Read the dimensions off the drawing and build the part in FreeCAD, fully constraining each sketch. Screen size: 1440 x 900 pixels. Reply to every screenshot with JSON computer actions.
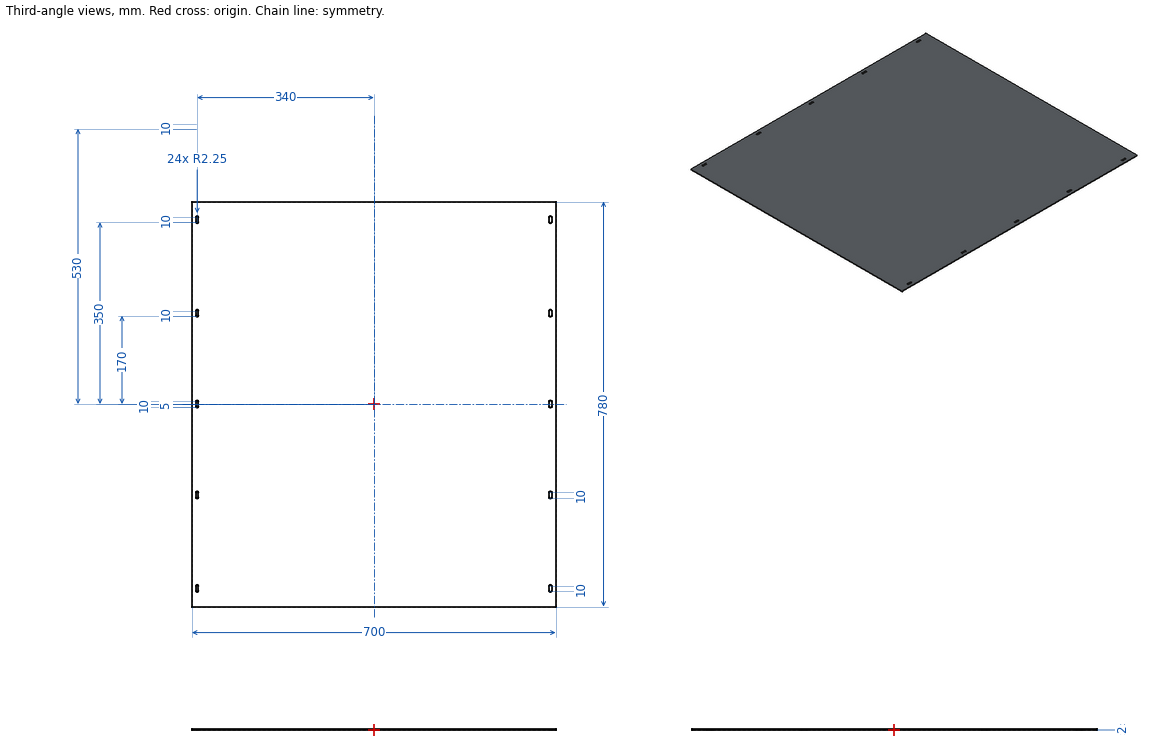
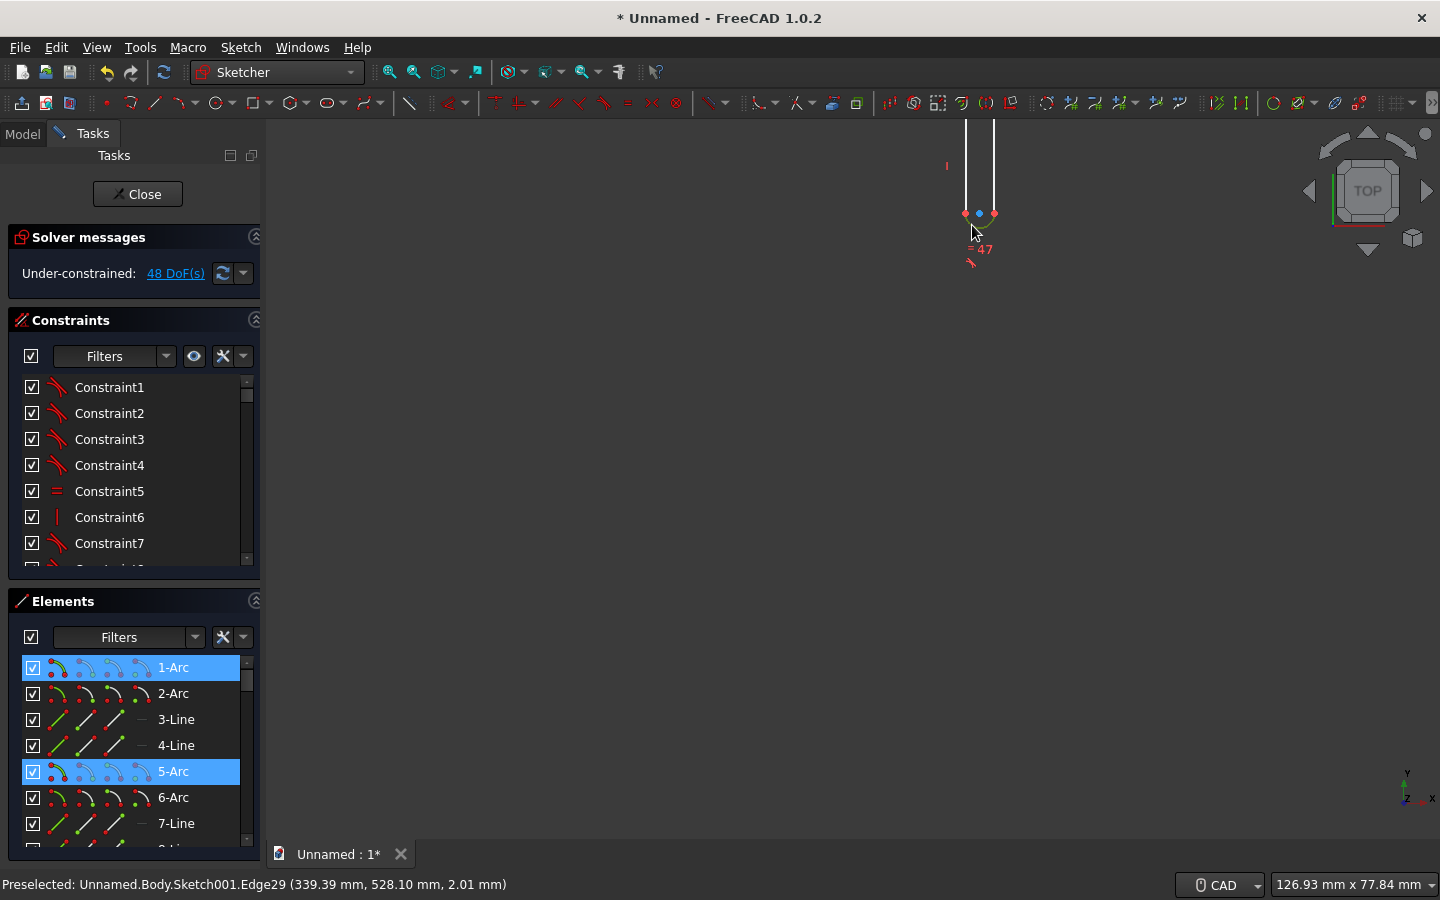
{"action": "scroll", "coordinate": [976, 233], "scroll_direction": "down", "scroll_amount": 14}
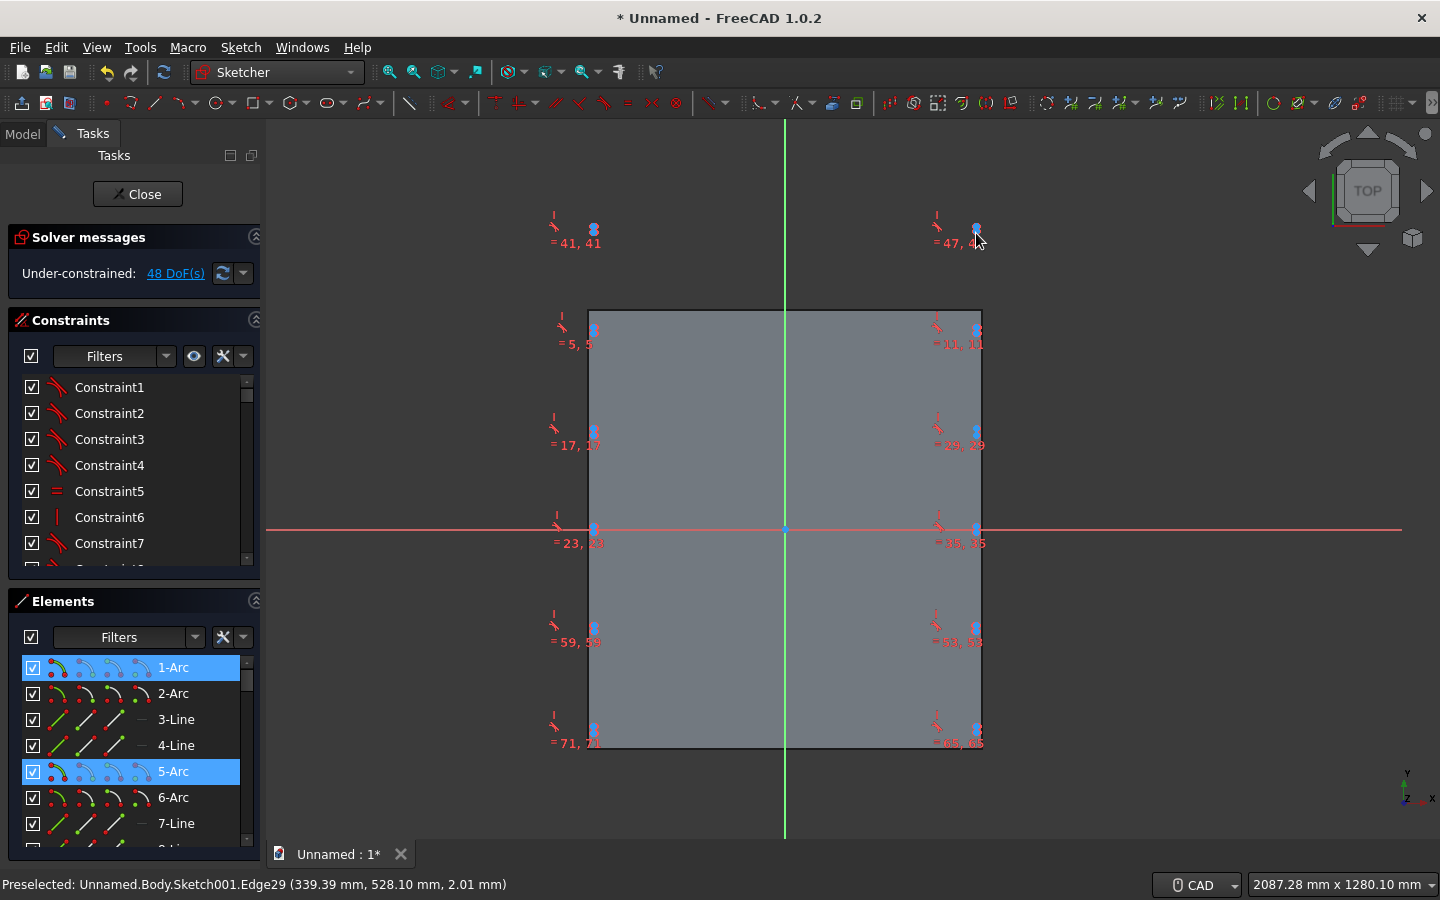
{"action": "scroll", "coordinate": [976, 633], "scroll_direction": "up", "scroll_amount": 13}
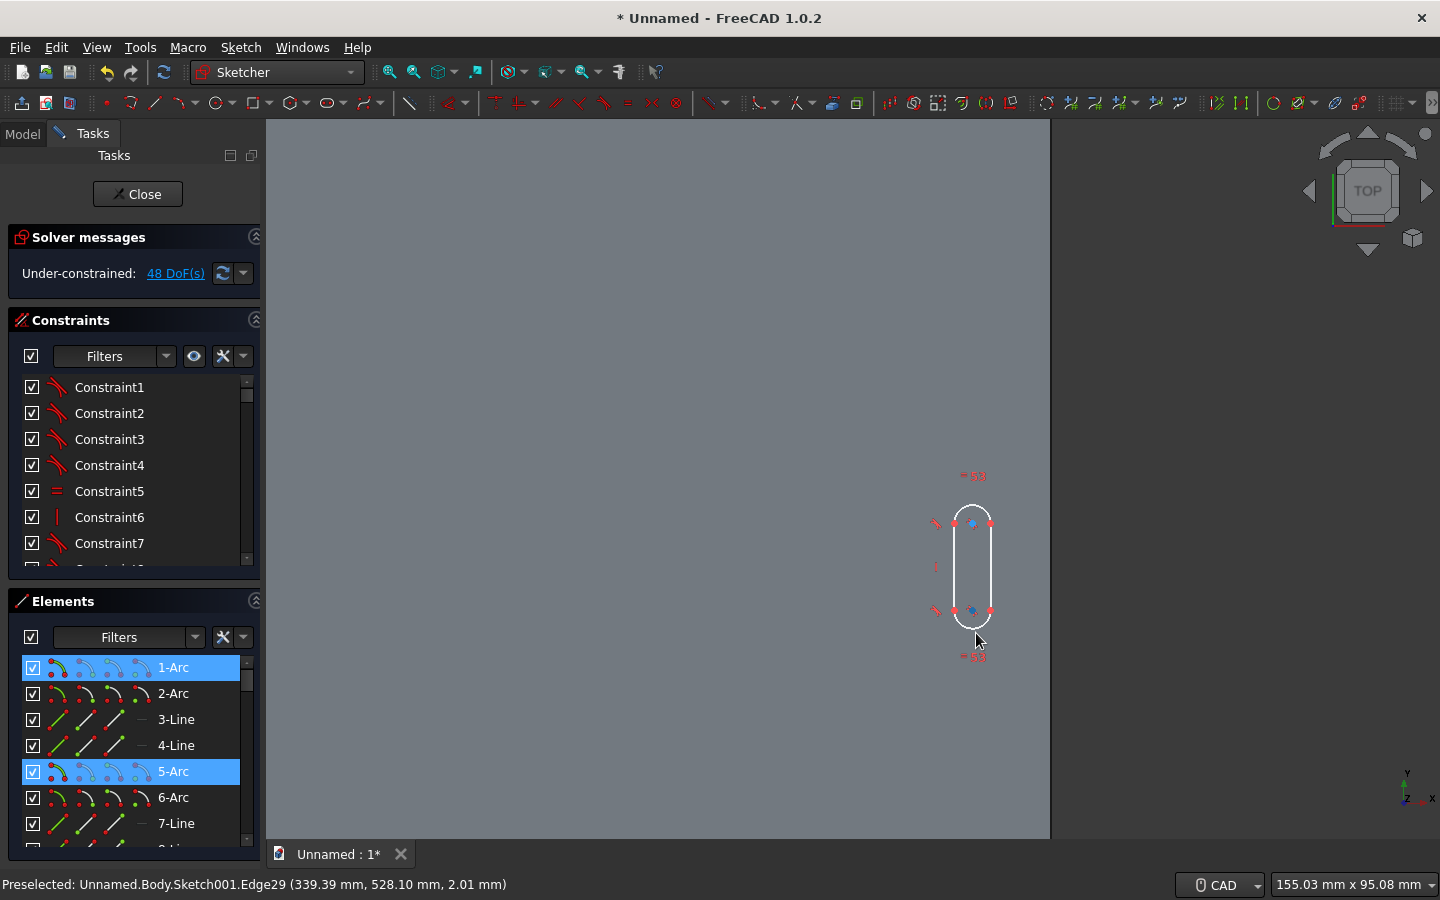
{"action": "left_click", "coordinate": [962, 625]}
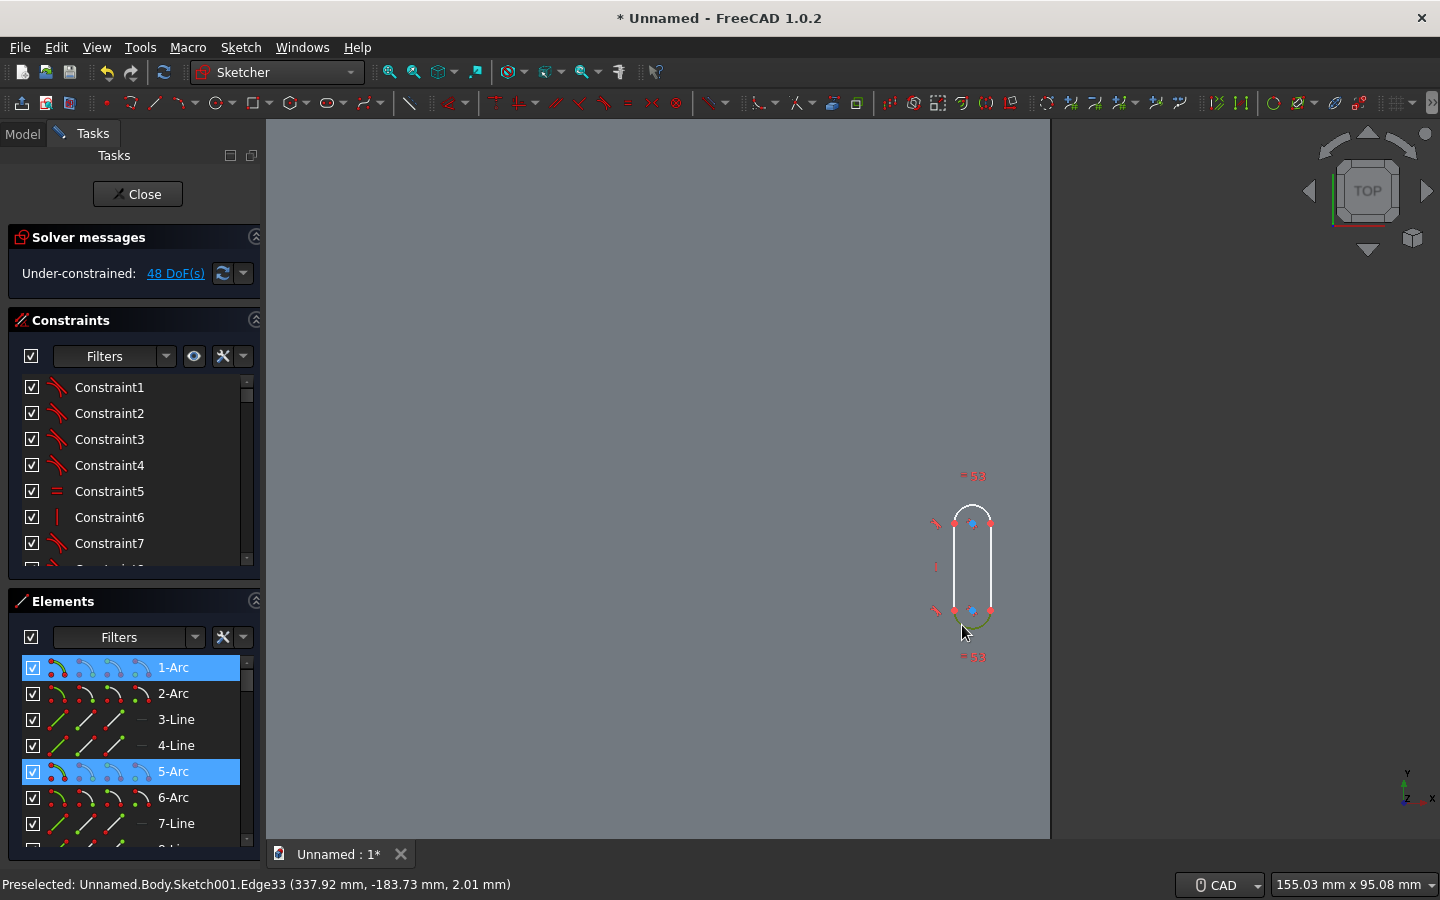
{"action": "scroll", "coordinate": [976, 634], "scroll_direction": "down", "scroll_amount": 13}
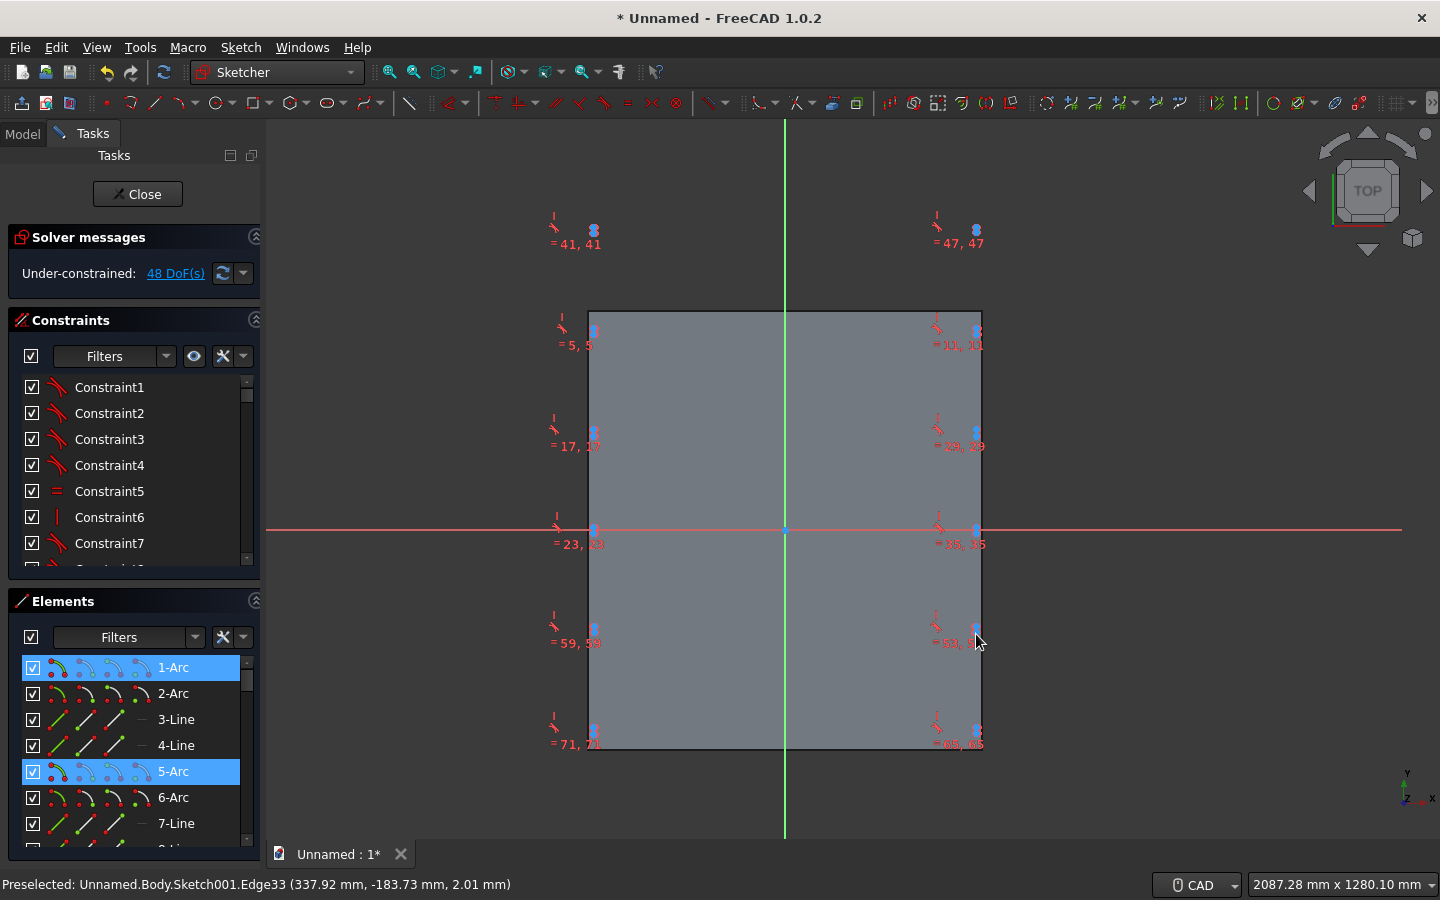
{"action": "scroll", "coordinate": [593, 634], "scroll_direction": "up", "scroll_amount": 12}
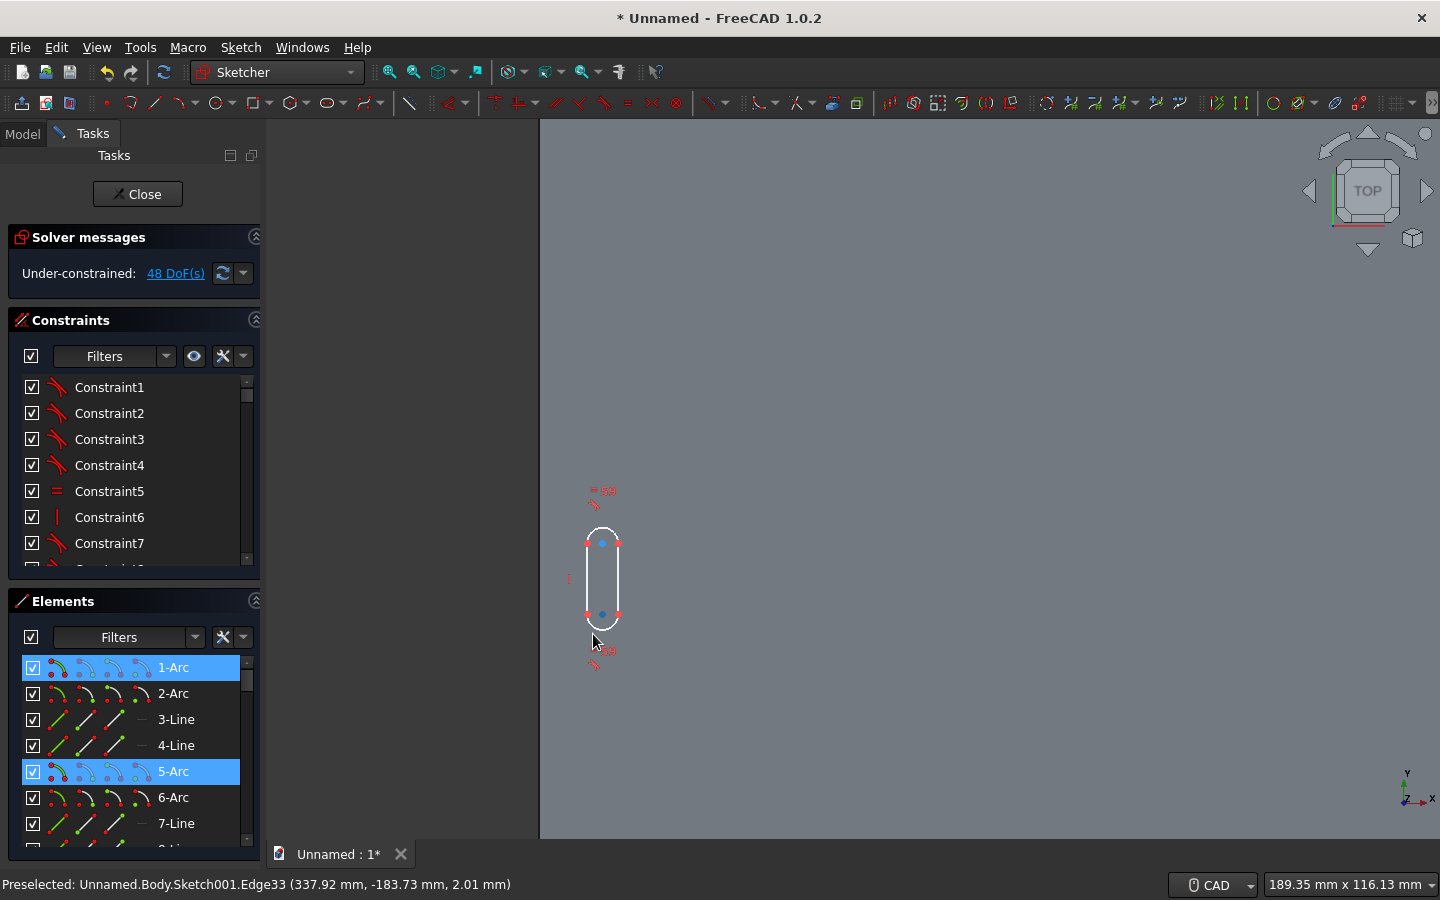
{"action": "left_click", "coordinate": [594, 627]}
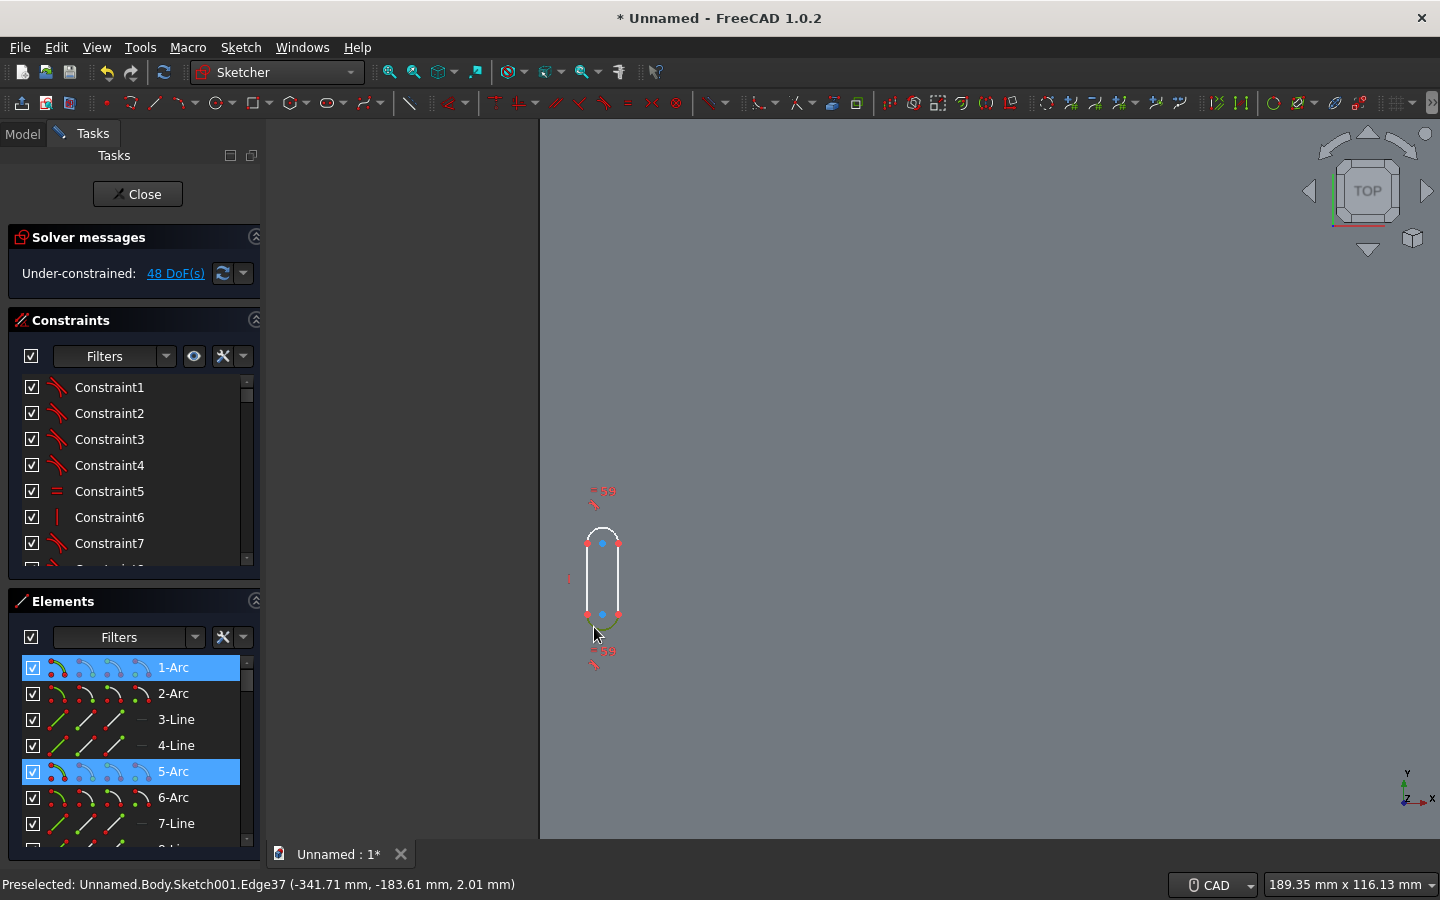
{"action": "scroll", "coordinate": [592, 634], "scroll_direction": "down", "scroll_amount": 12}